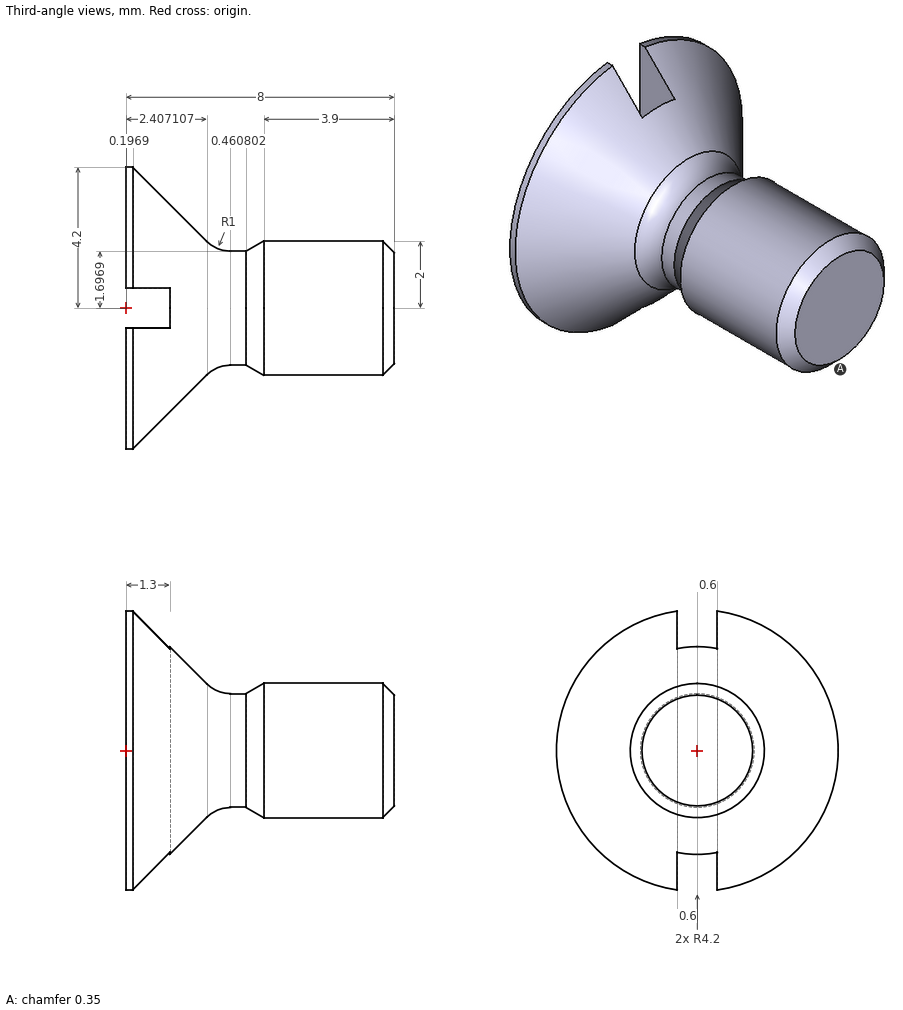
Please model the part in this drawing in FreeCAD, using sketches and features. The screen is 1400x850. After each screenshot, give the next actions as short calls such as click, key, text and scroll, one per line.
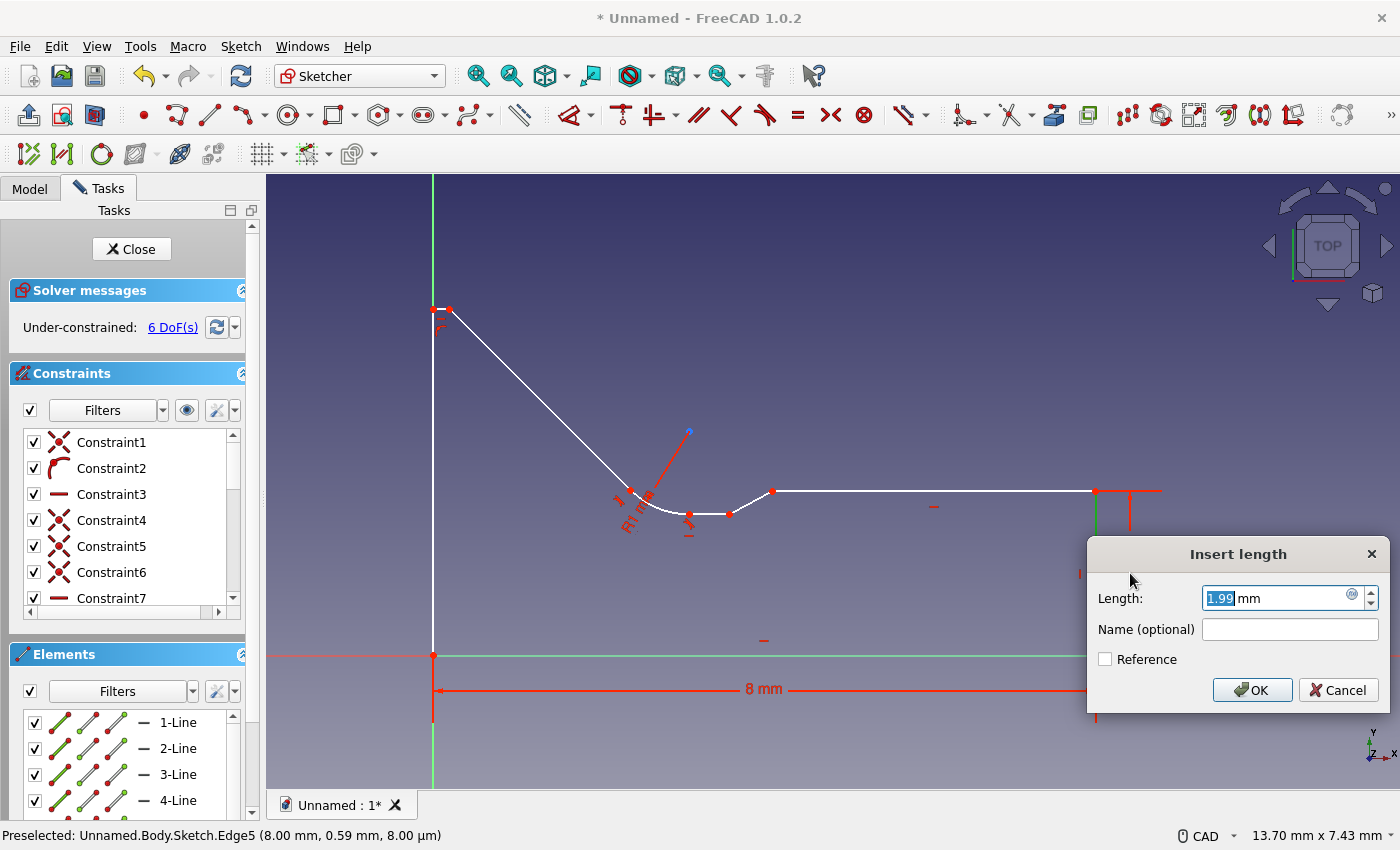
text(2)
key(Return)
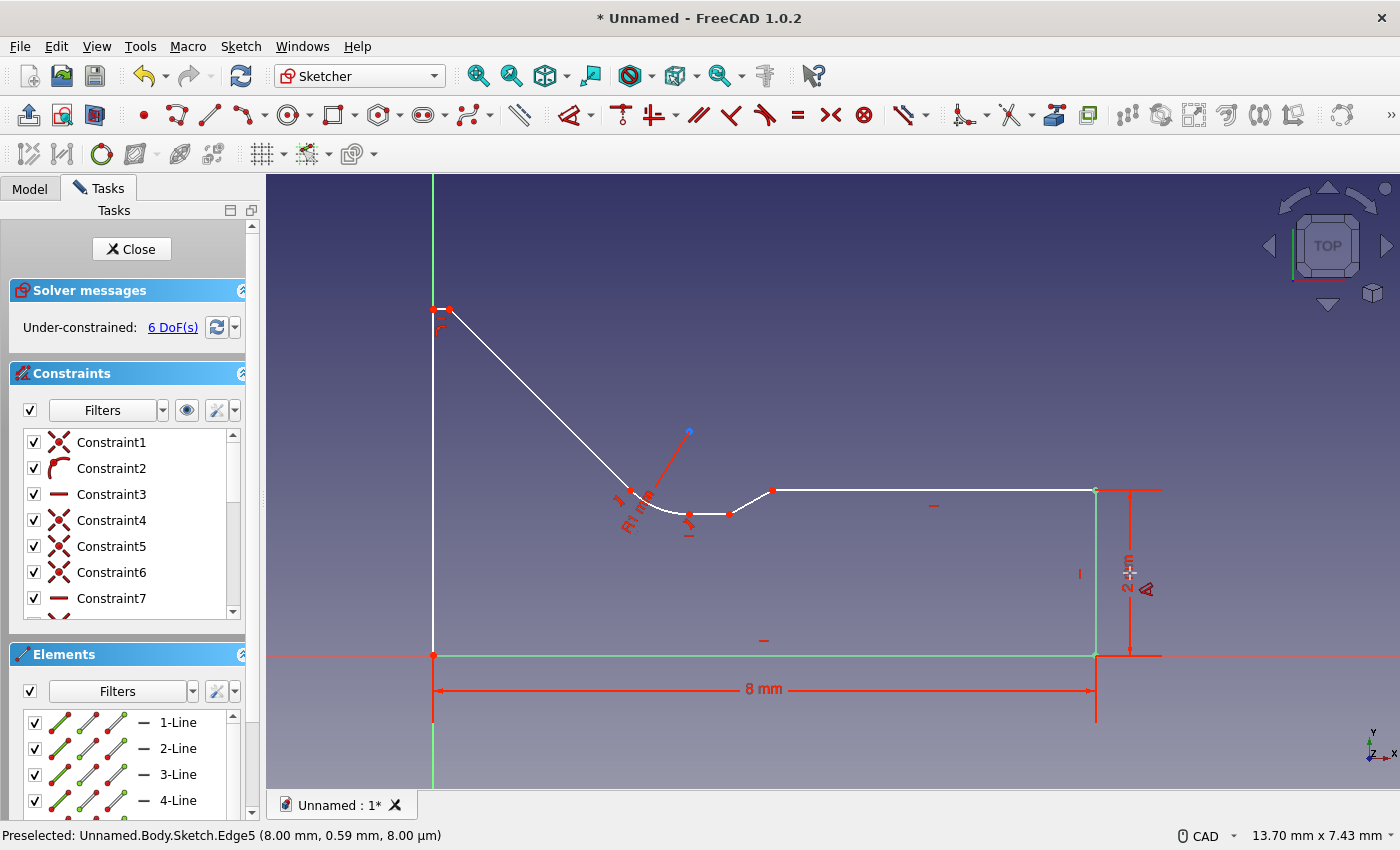
click(433, 413)
click(399, 482)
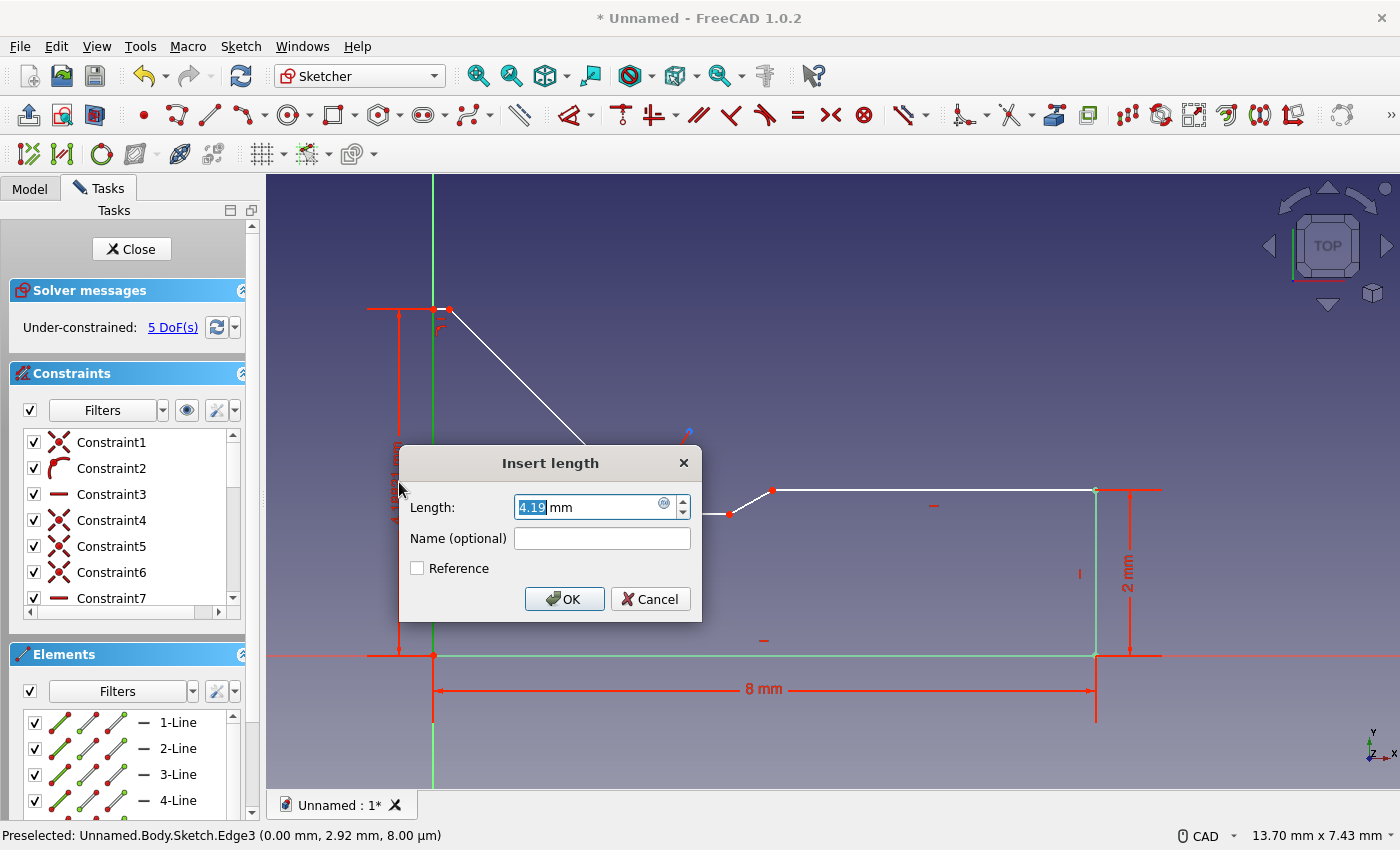
text(4.2)
key(Return)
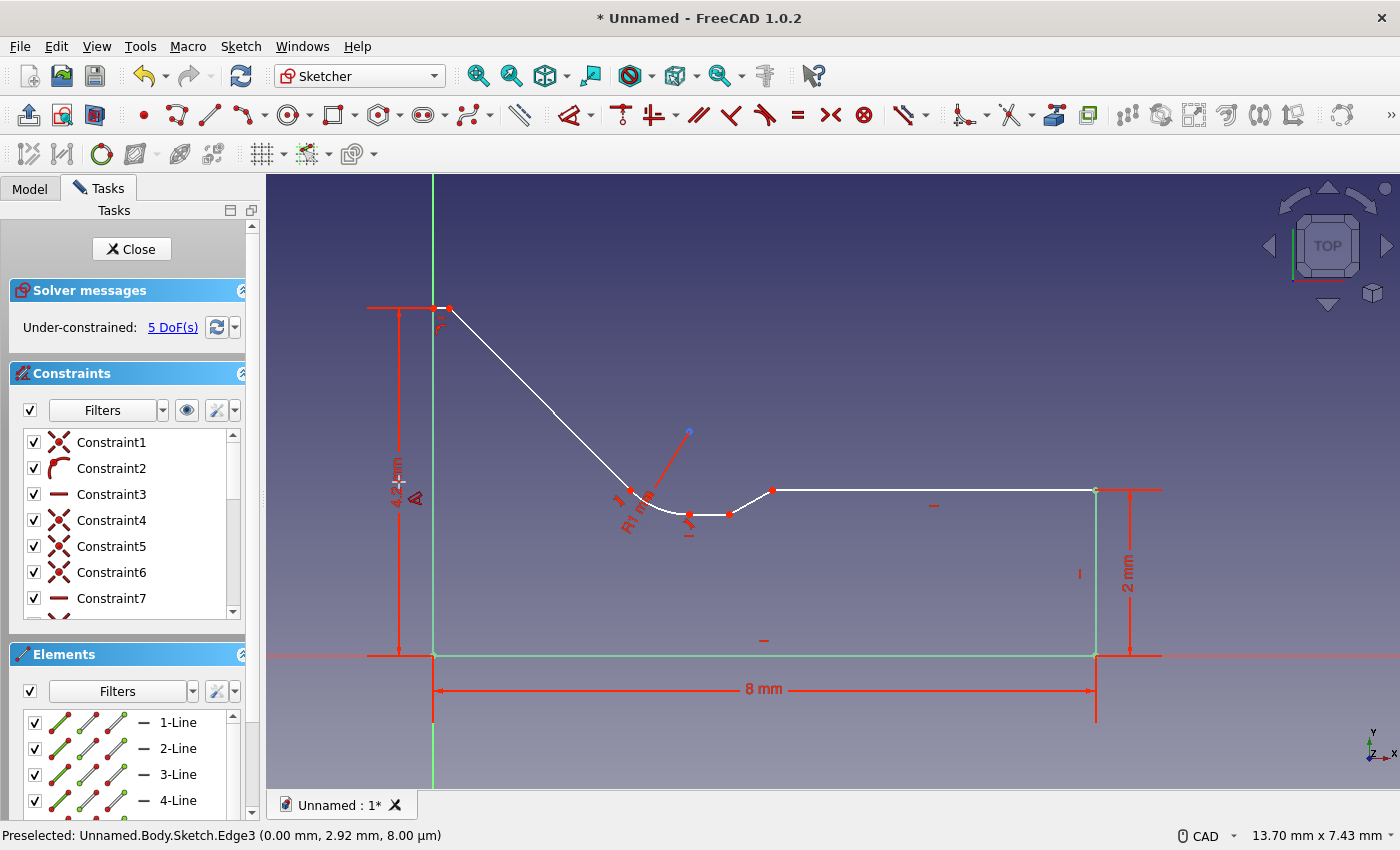
click(999, 490)
click(934, 524)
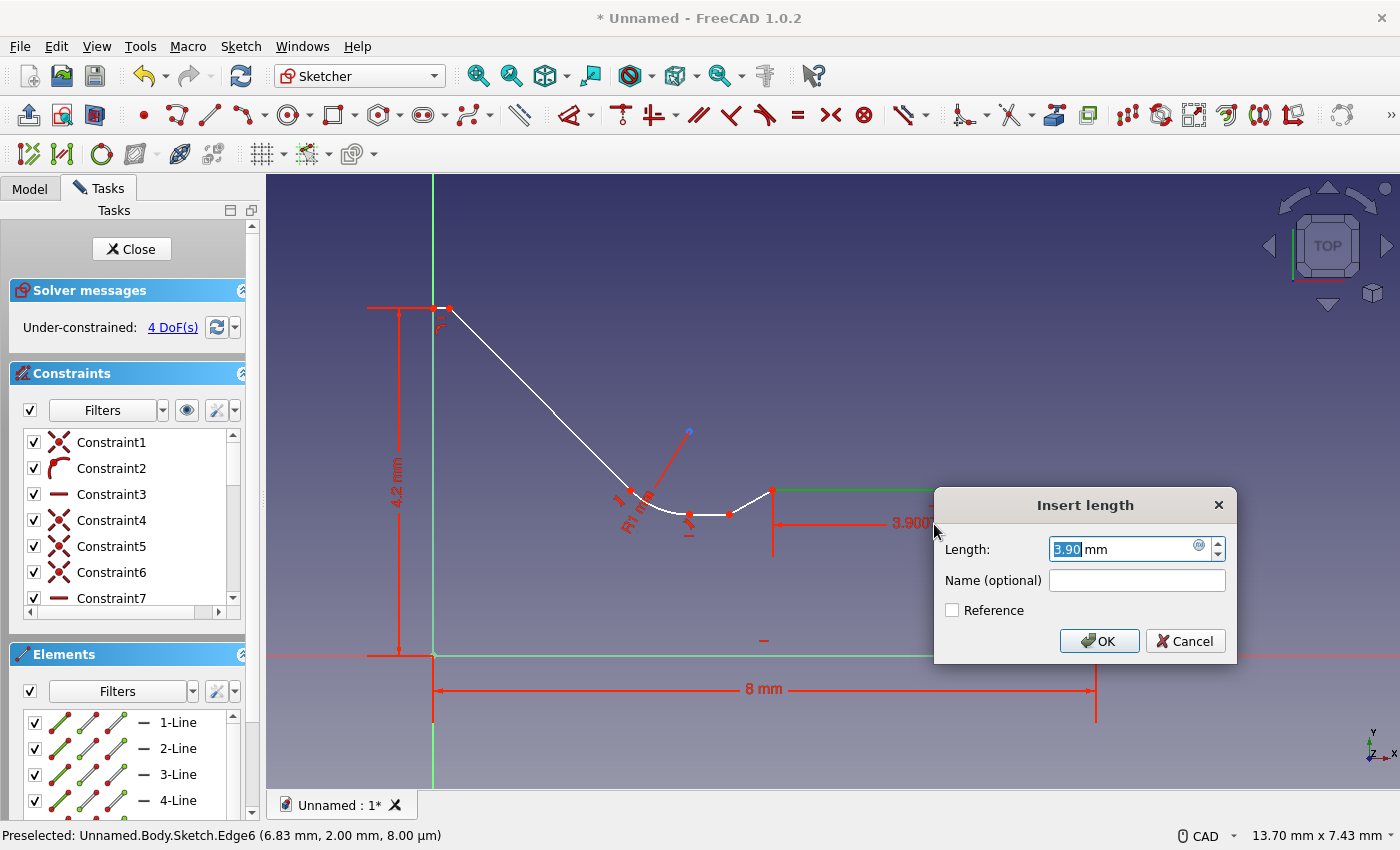
text(3.9)
key(Return)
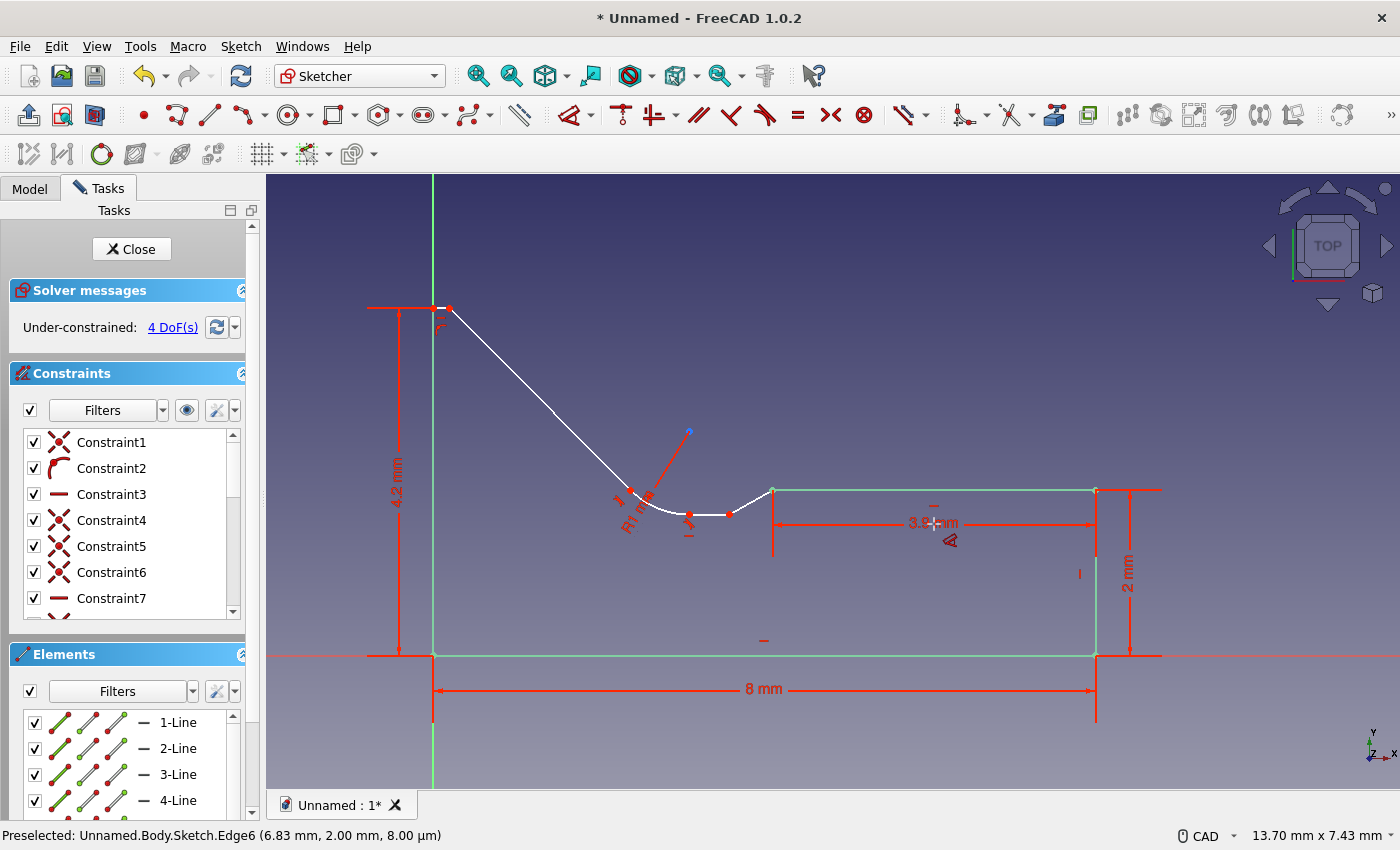
scroll(441, 308, up, 5)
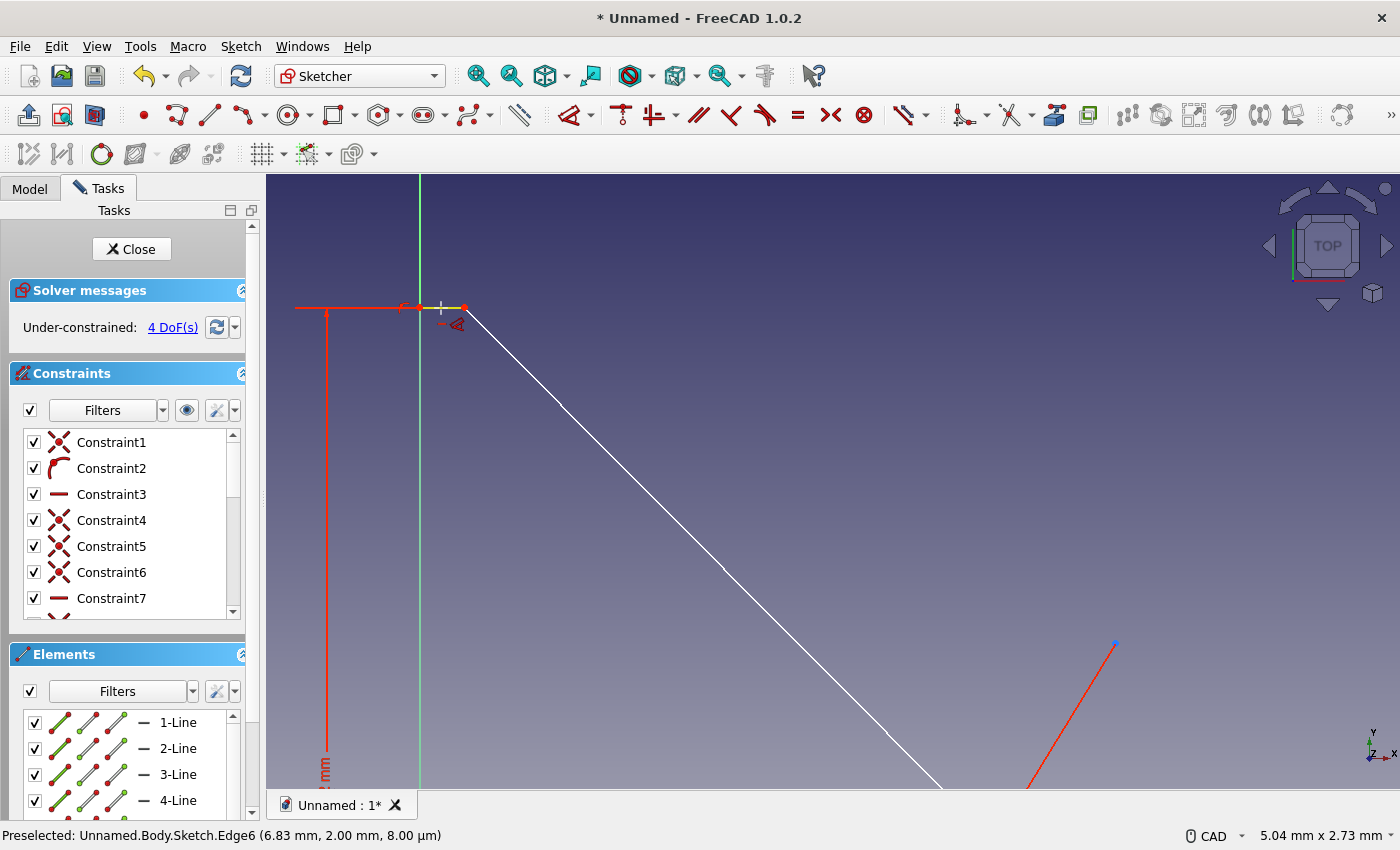
click(442, 308)
click(442, 274)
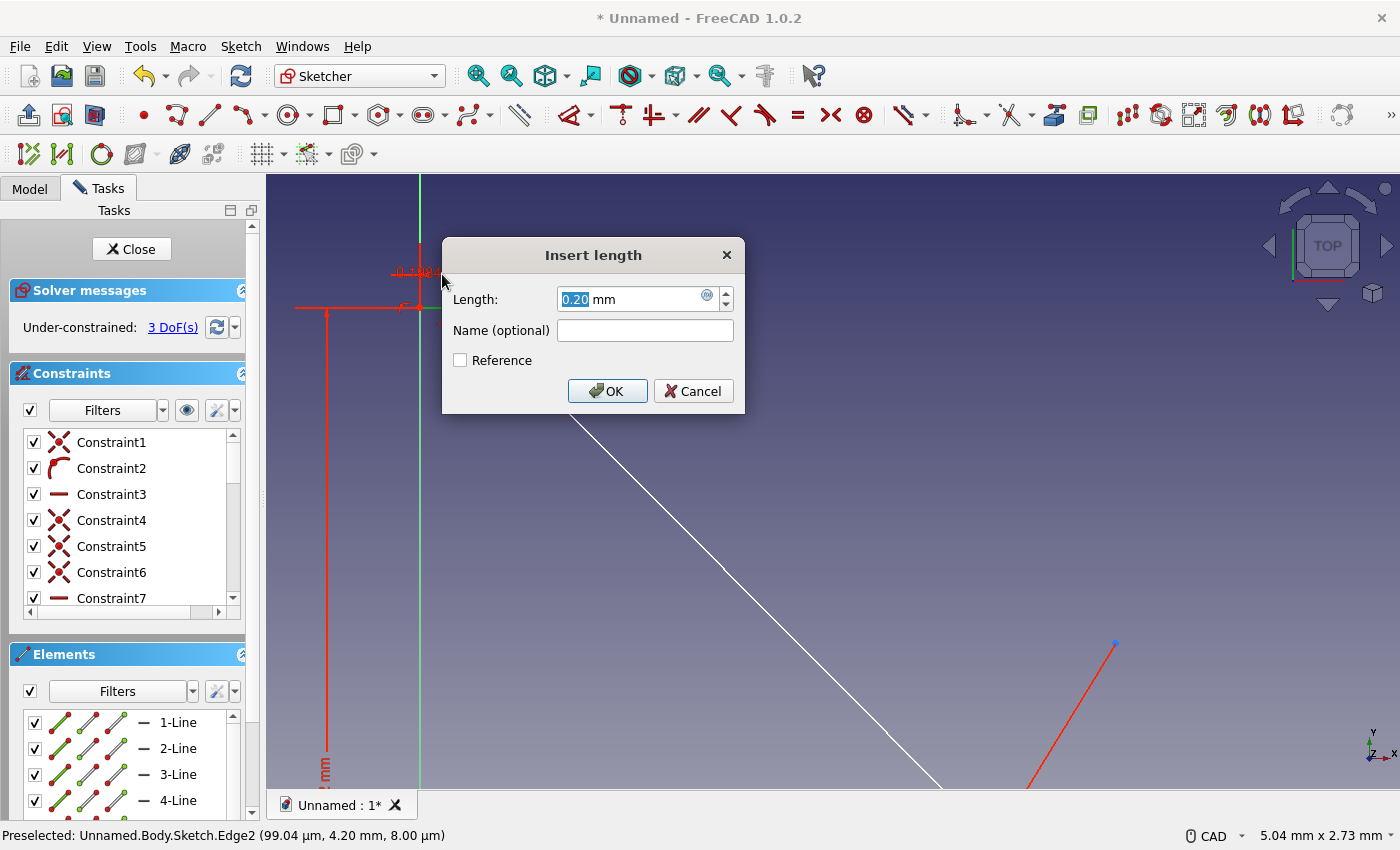
text(0.1969)
key(Return)